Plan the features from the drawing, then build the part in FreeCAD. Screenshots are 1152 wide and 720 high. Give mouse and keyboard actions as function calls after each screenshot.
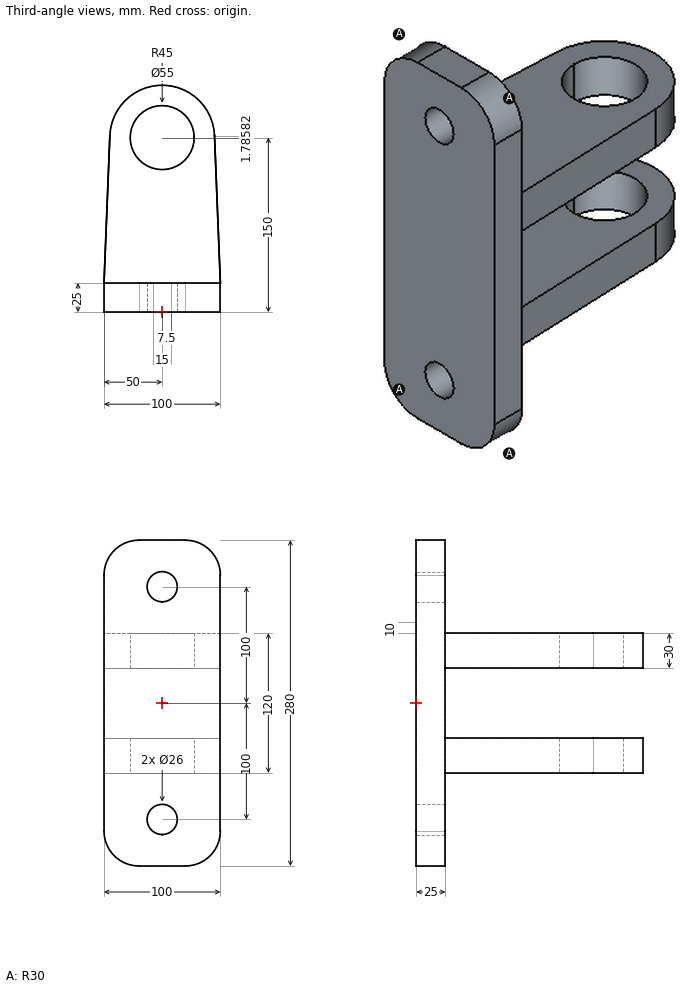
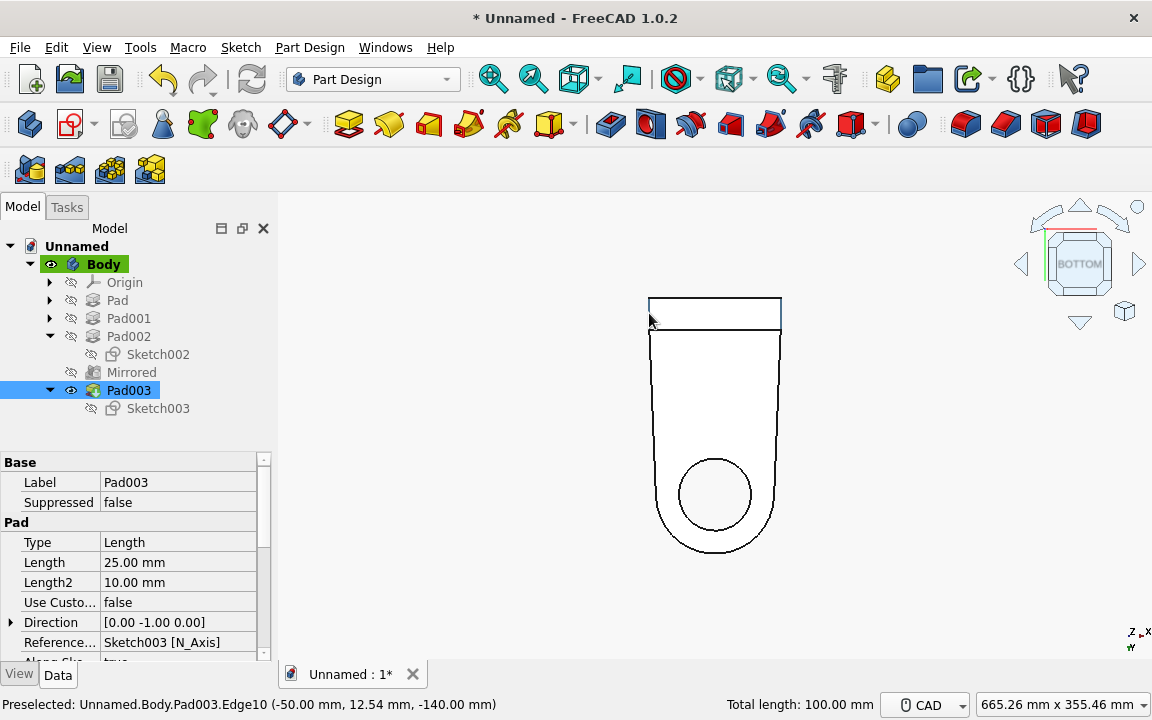
click(966, 124)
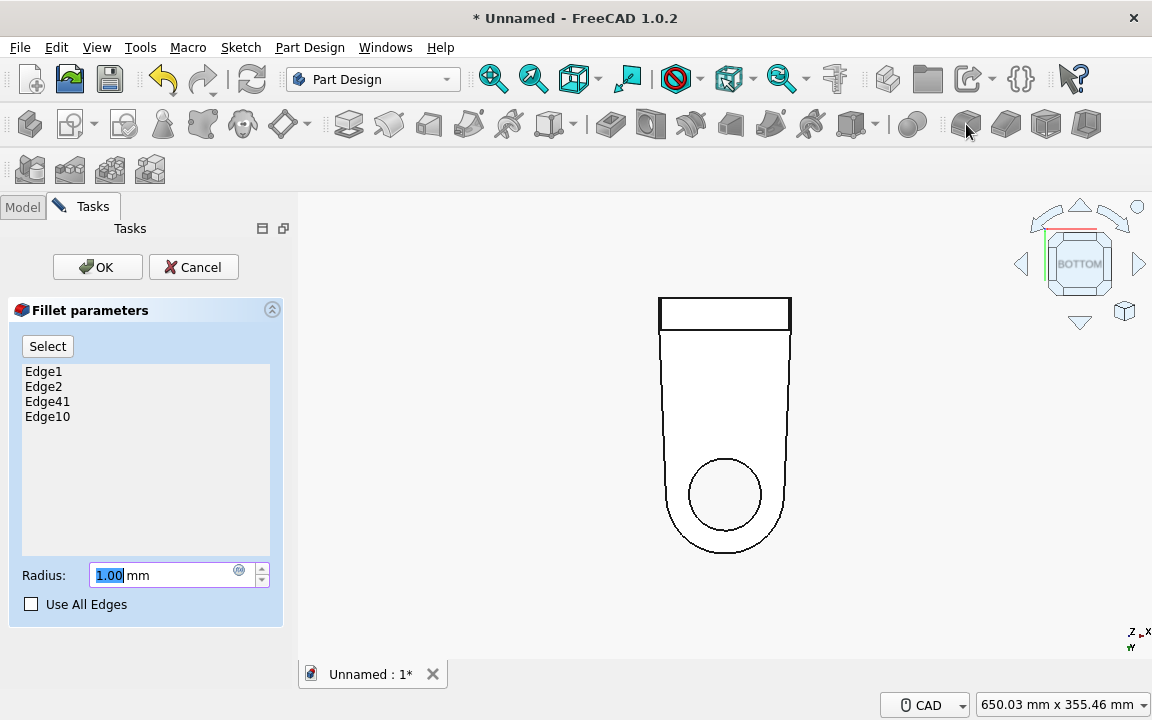
text(30)
key(Tab)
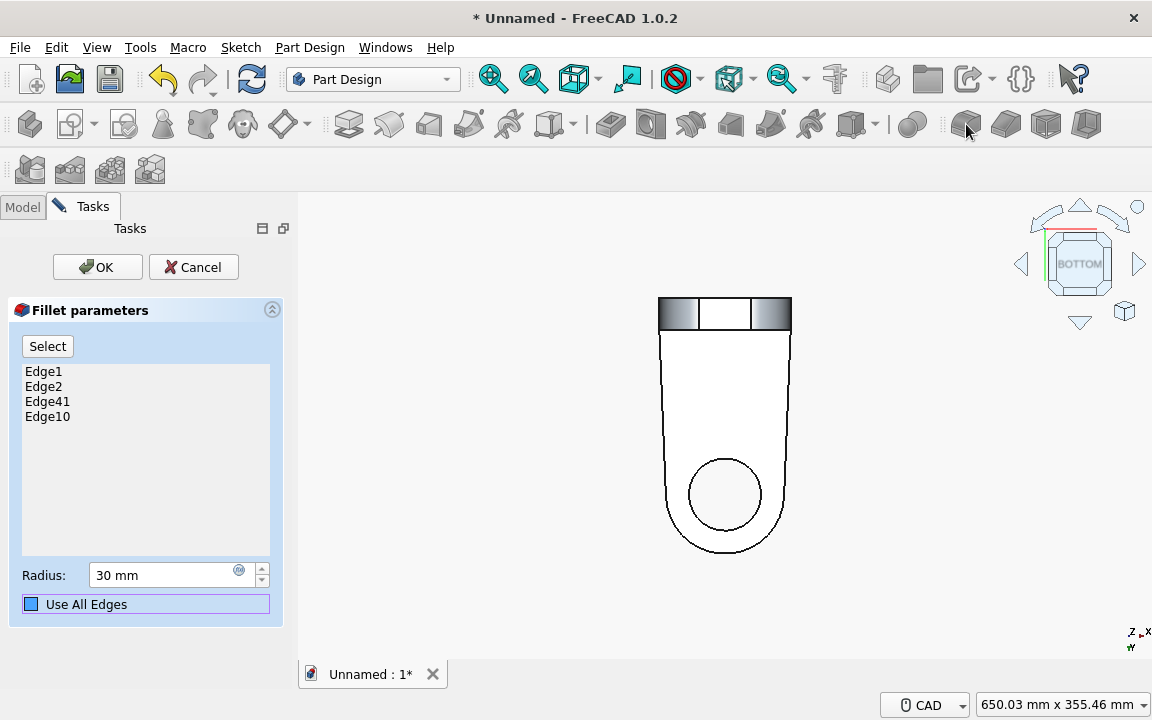
click(98, 267)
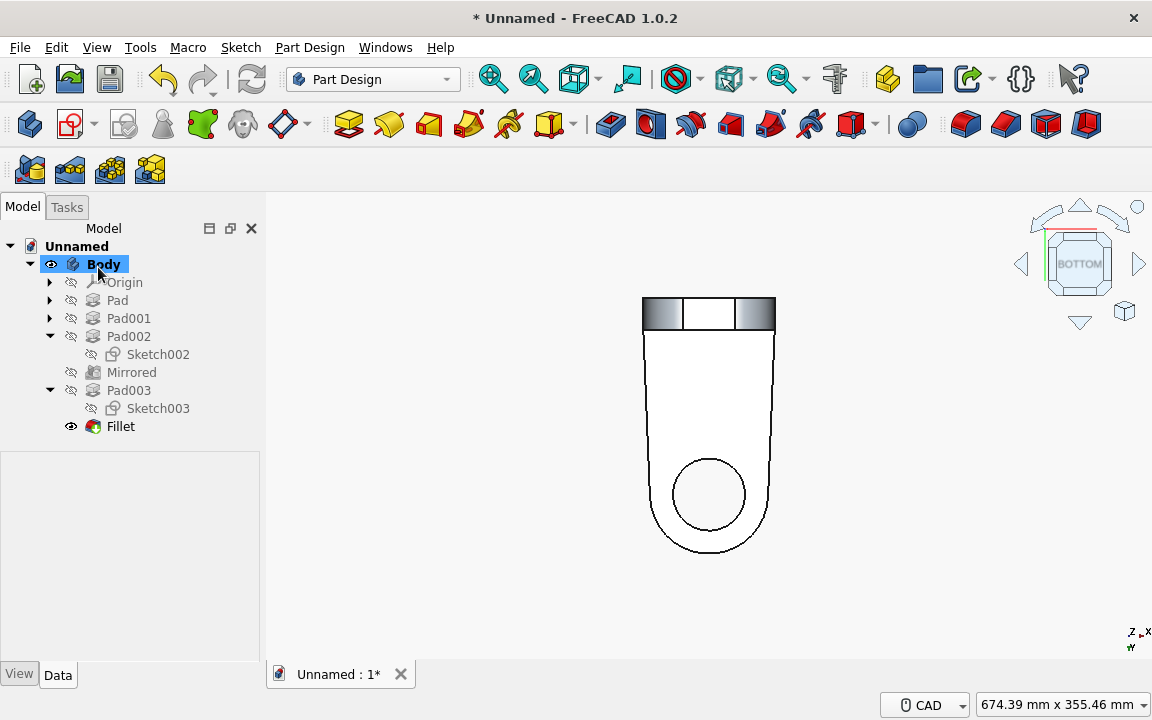
key(0)